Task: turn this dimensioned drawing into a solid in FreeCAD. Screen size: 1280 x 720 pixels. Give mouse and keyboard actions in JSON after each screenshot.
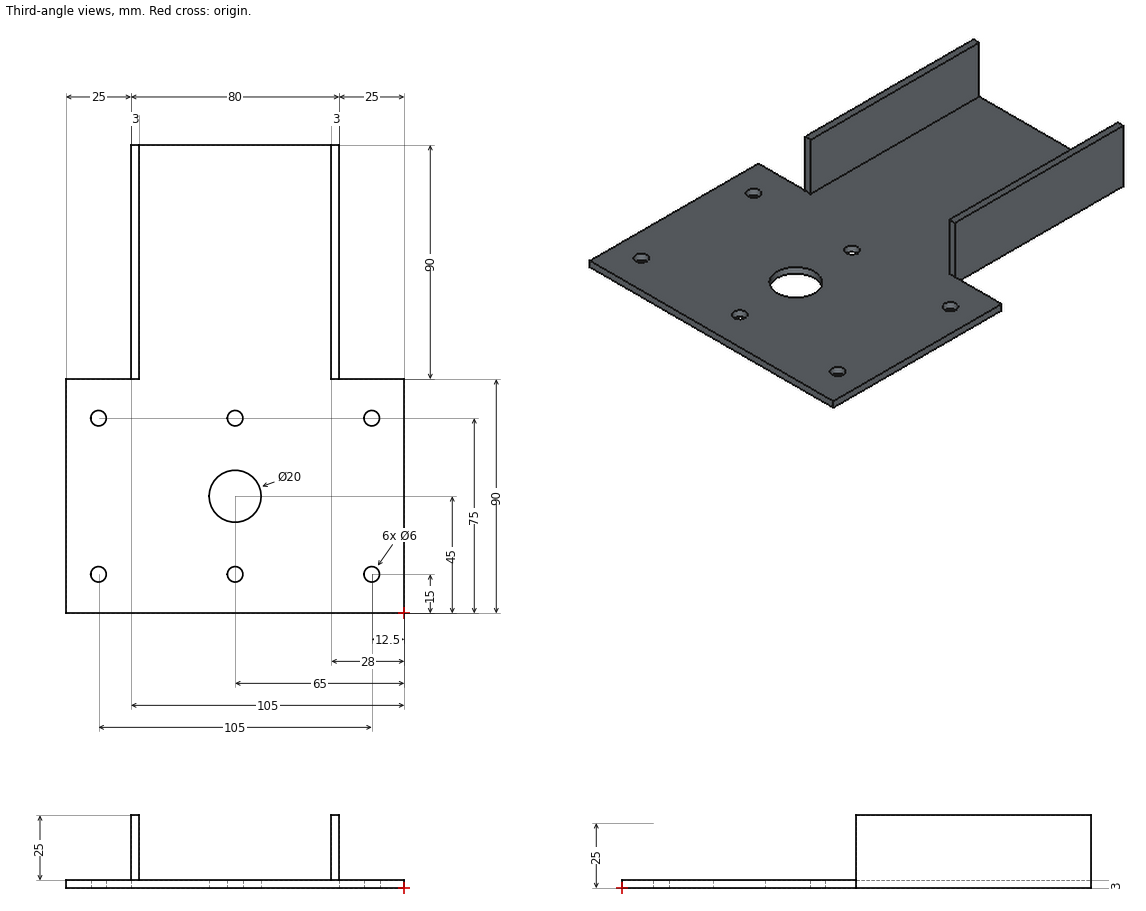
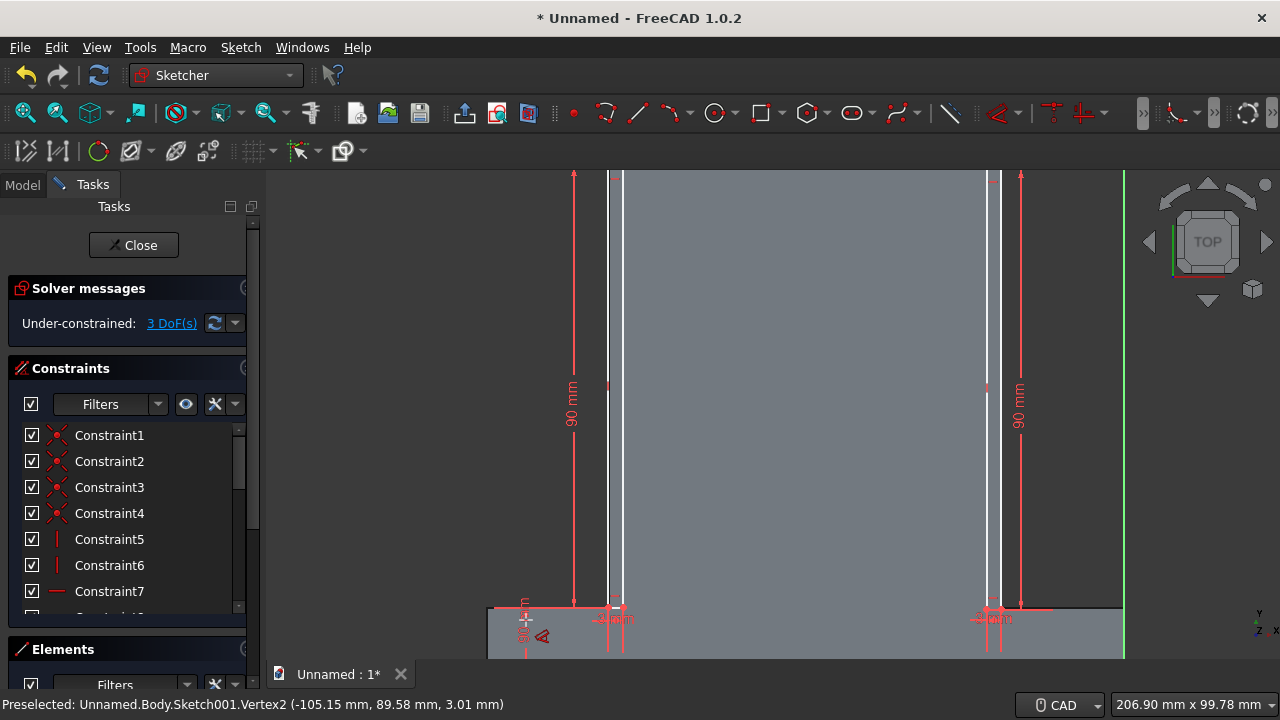
{"action": "scroll", "coordinate": [610, 302], "scroll_direction": "down", "scroll_amount": 5}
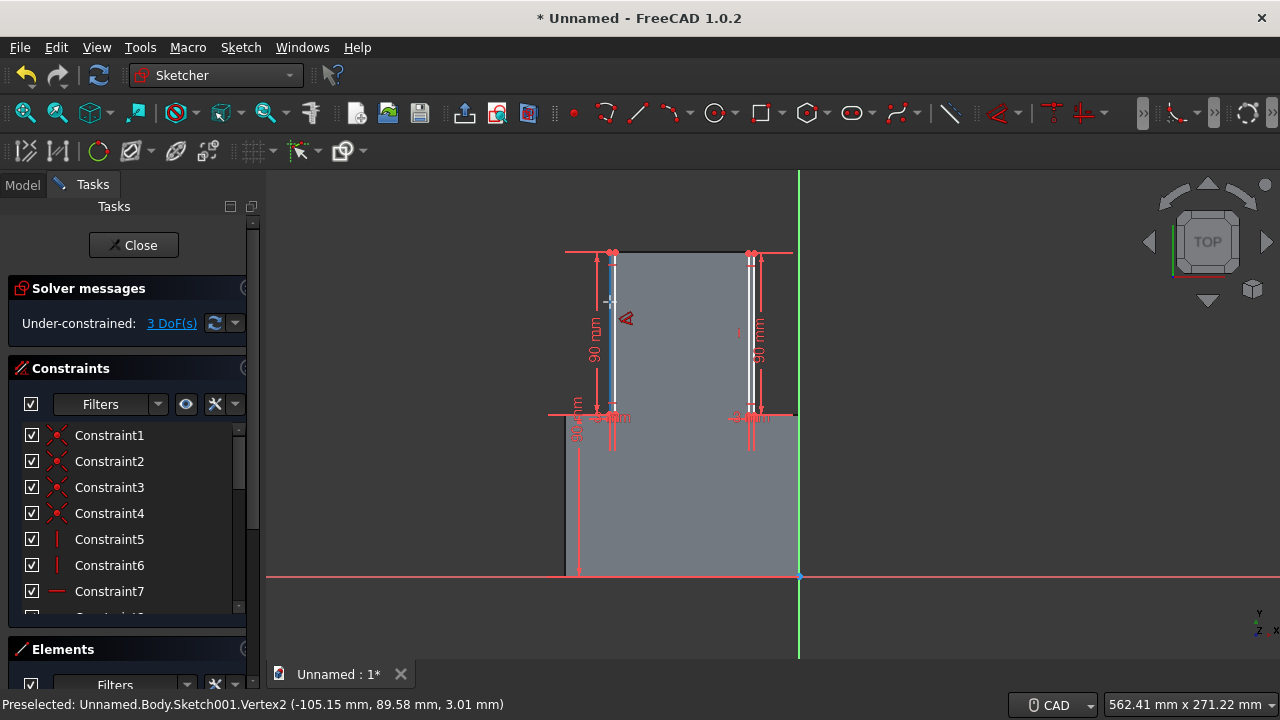
{"action": "scroll", "coordinate": [749, 253], "scroll_direction": "up", "scroll_amount": 5}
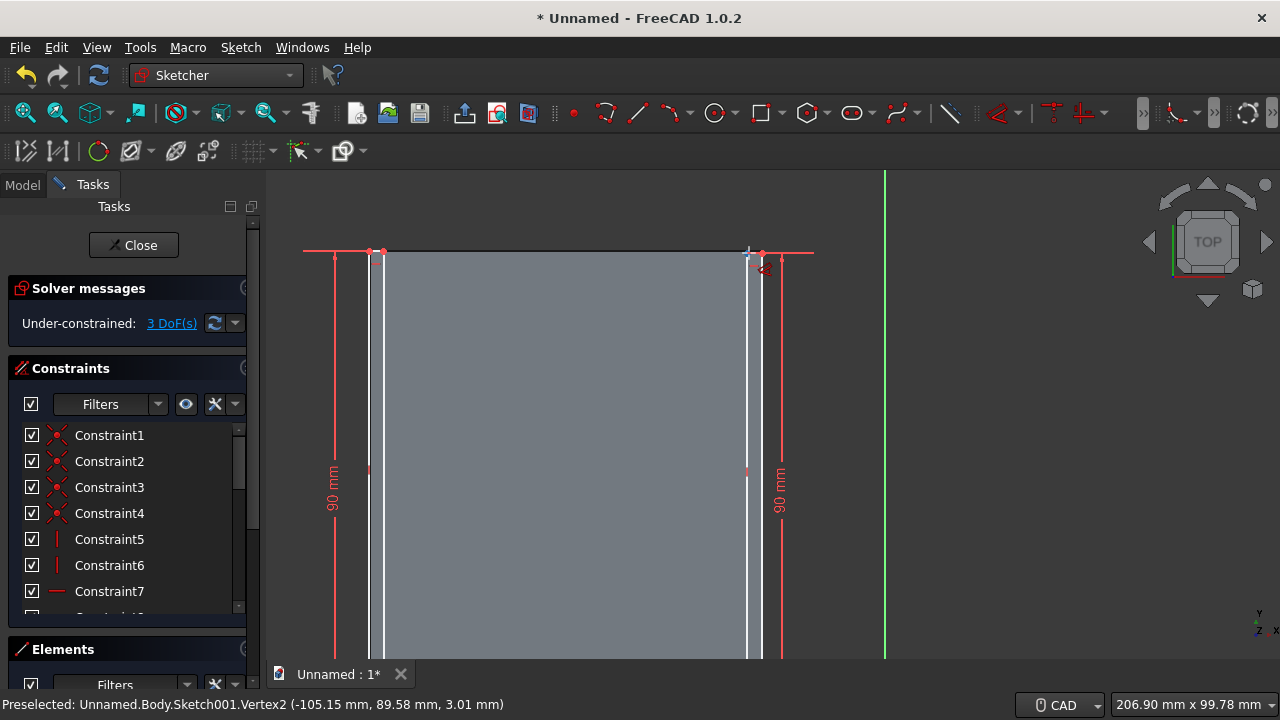
{"action": "left_click", "coordinate": [747, 253]}
{"action": "left_click", "coordinate": [816, 219]}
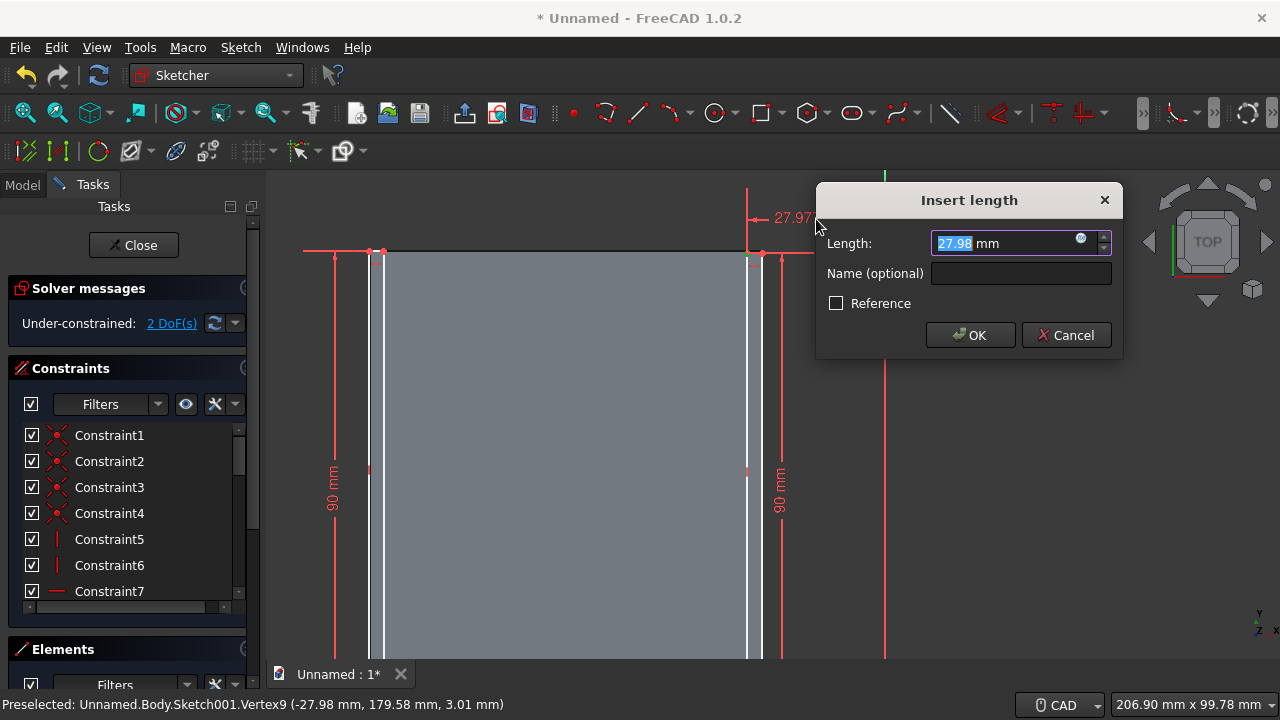
{"action": "type", "text": "28"}
{"action": "key", "text": "Return"}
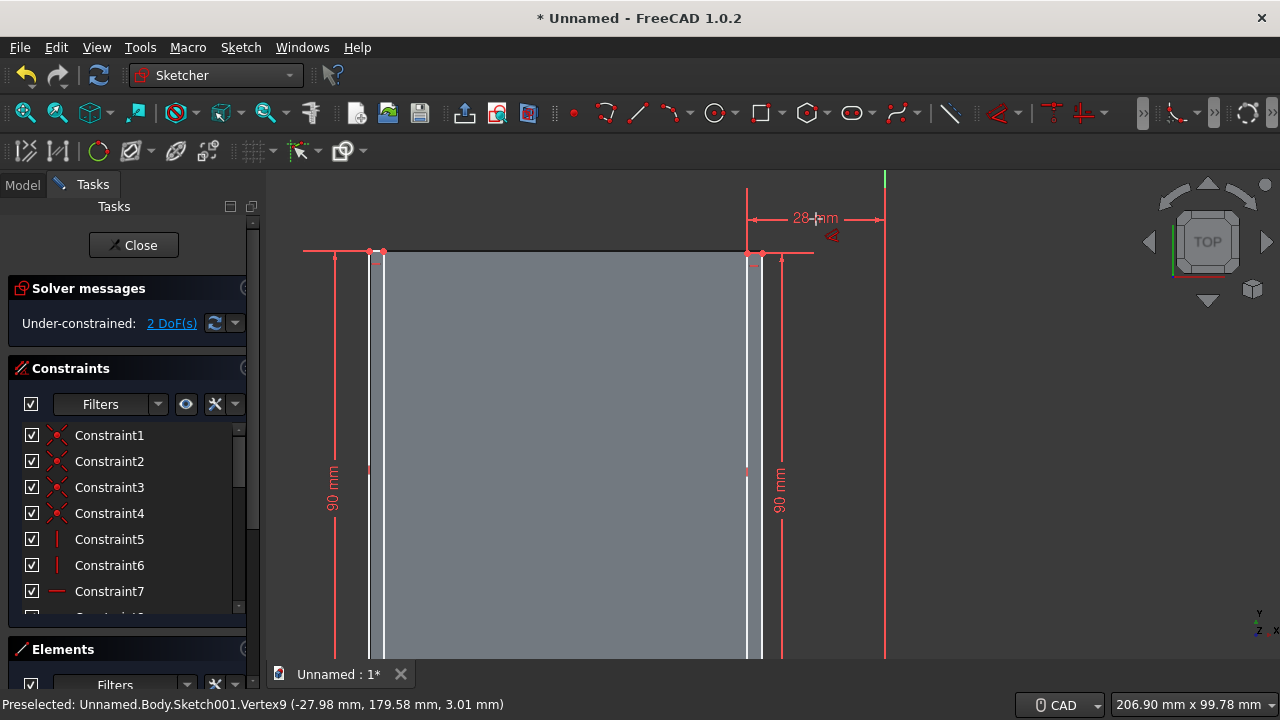
{"action": "scroll", "coordinate": [749, 253], "scroll_direction": "down", "scroll_amount": 5}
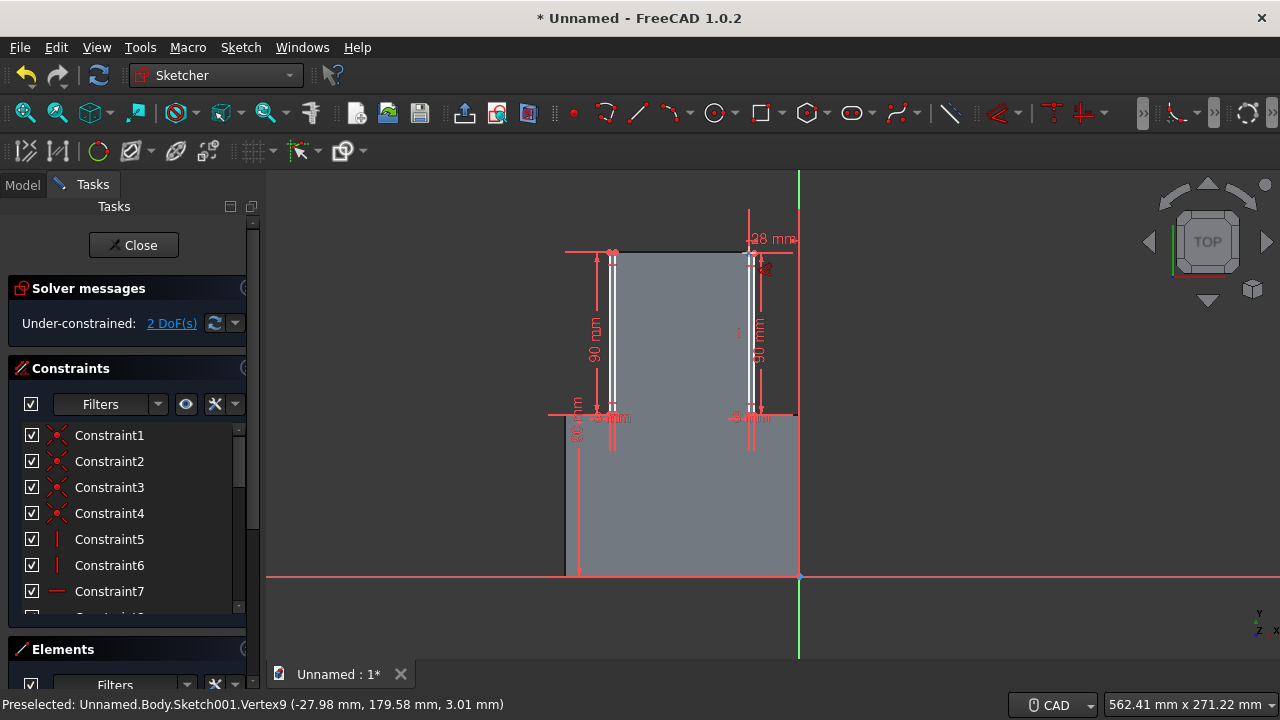
{"action": "scroll", "coordinate": [749, 415], "scroll_direction": "up", "scroll_amount": 5}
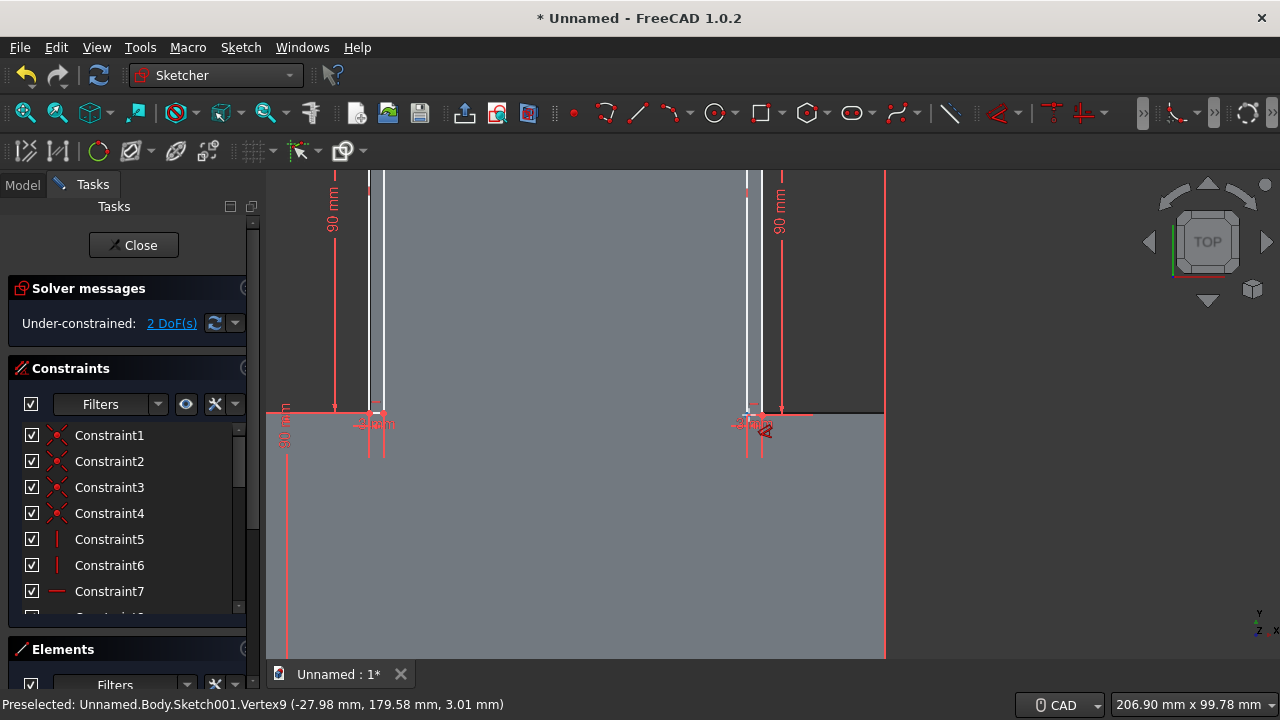
{"action": "left_click", "coordinate": [747, 415]}
{"action": "left_click", "coordinate": [919, 523]}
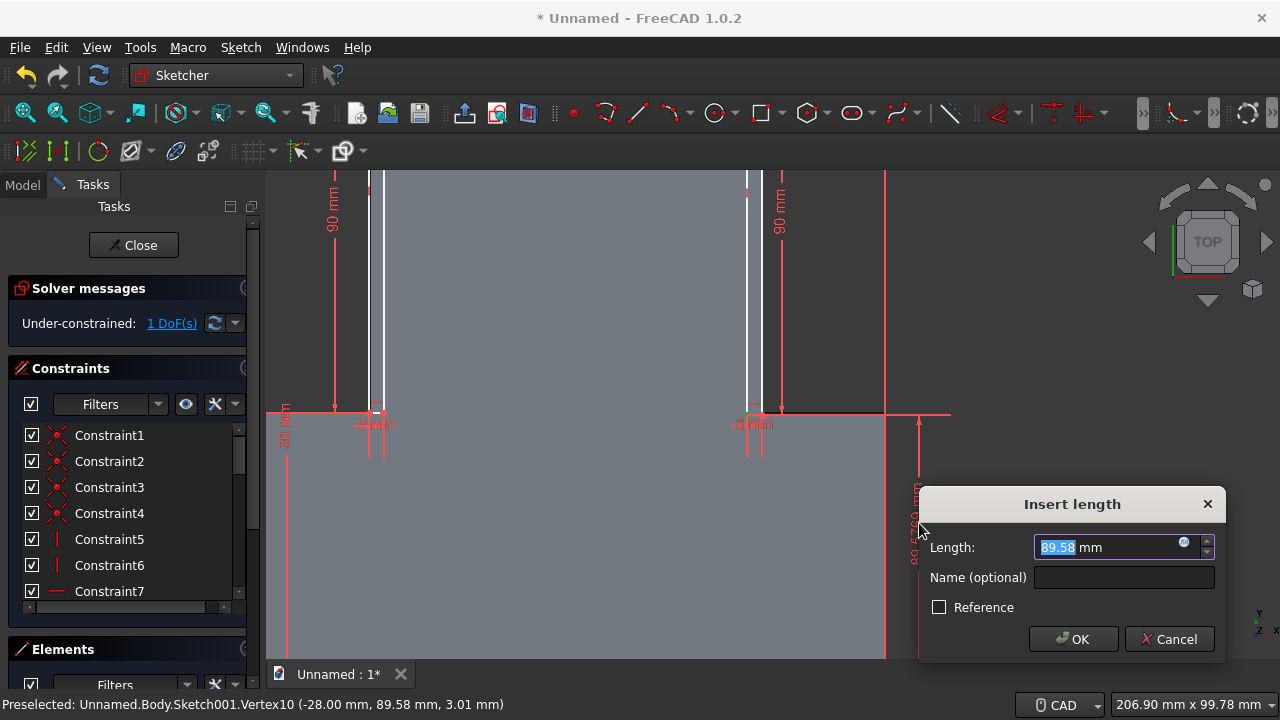
{"action": "type", "text": "90"}
{"action": "key", "text": "Return"}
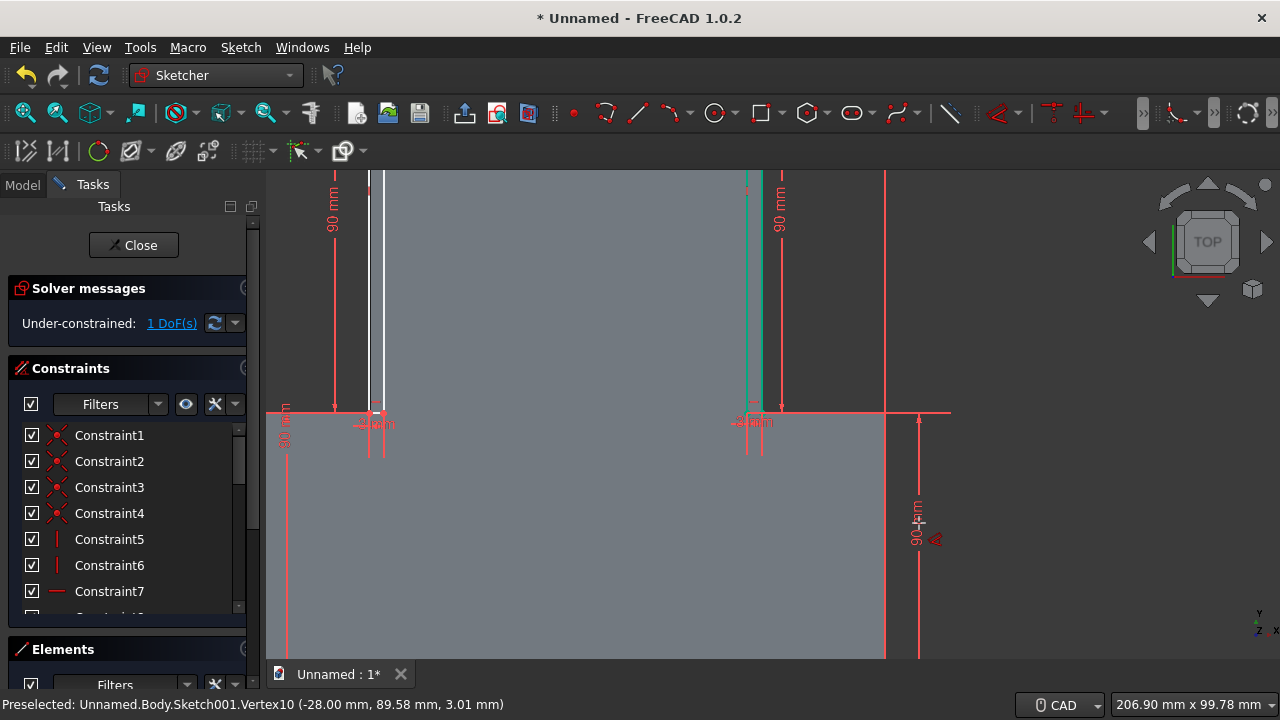
{"action": "scroll", "coordinate": [749, 415], "scroll_direction": "down", "scroll_amount": 5}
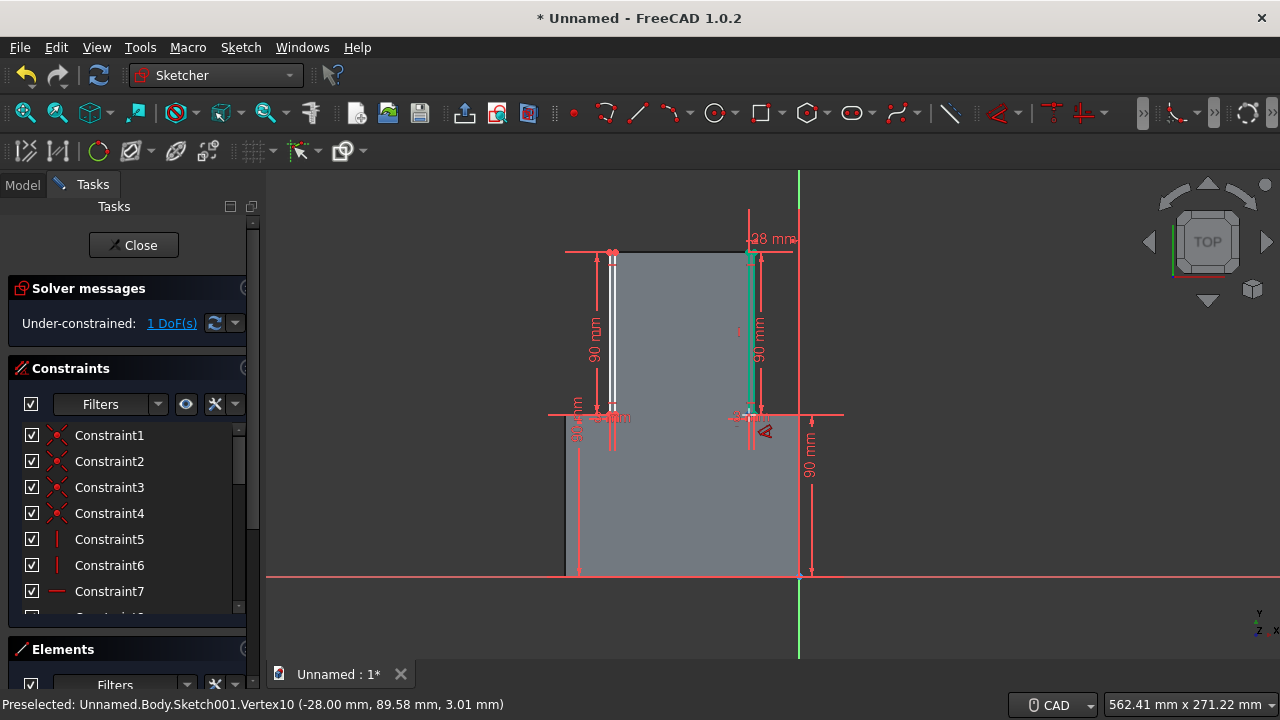
{"action": "scroll", "coordinate": [610, 252], "scroll_direction": "up", "scroll_amount": 5}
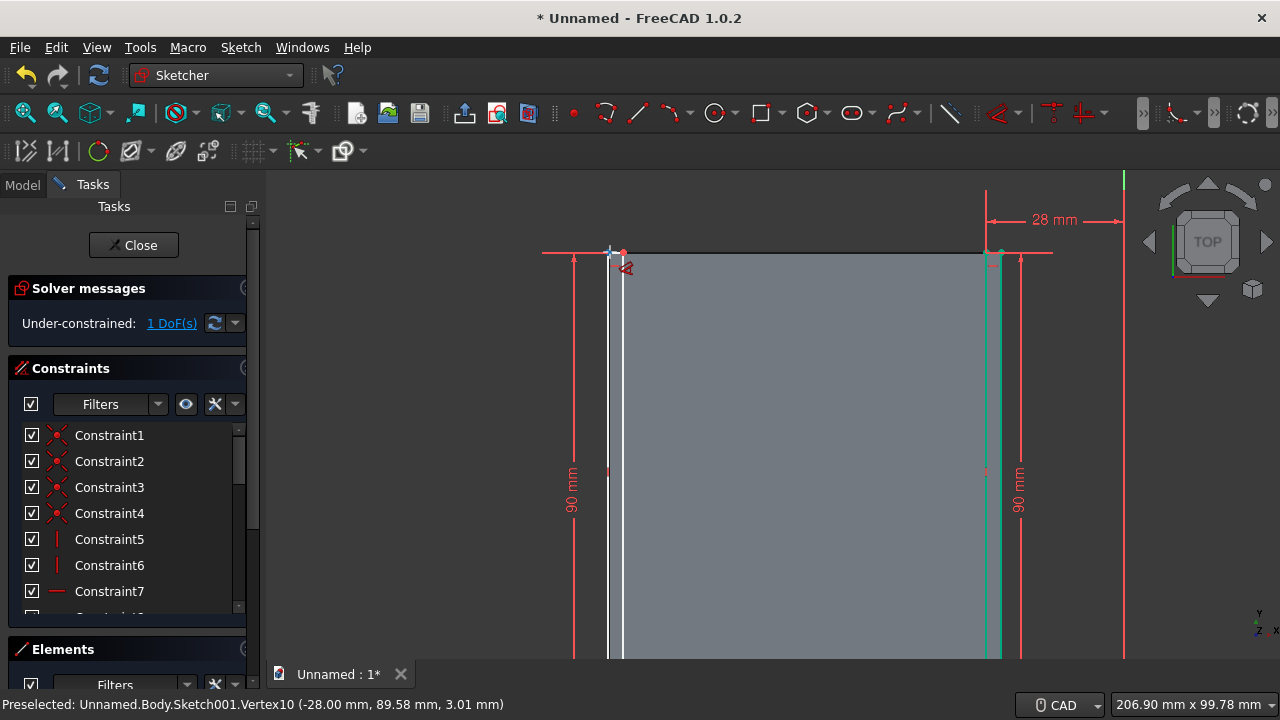
{"action": "left_click", "coordinate": [608, 253]}
{"action": "left_click", "coordinate": [862, 219]}